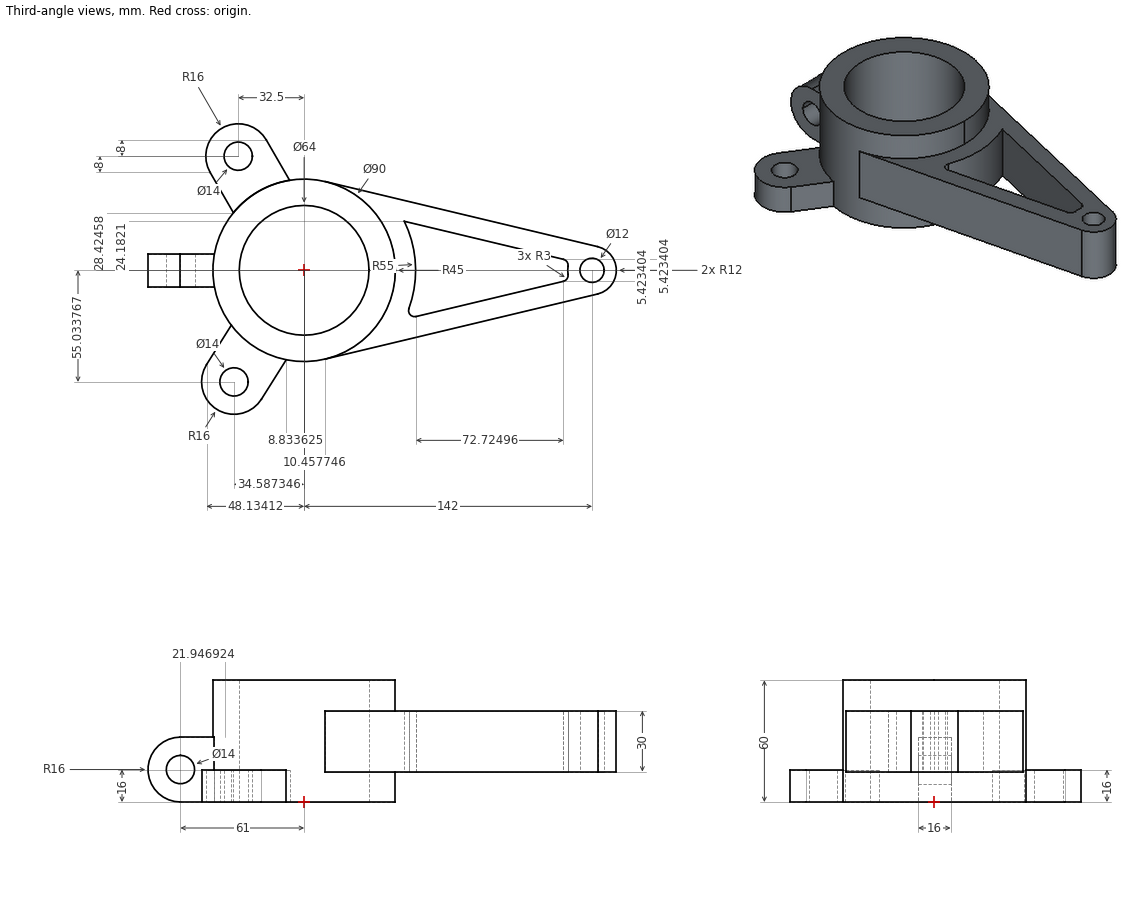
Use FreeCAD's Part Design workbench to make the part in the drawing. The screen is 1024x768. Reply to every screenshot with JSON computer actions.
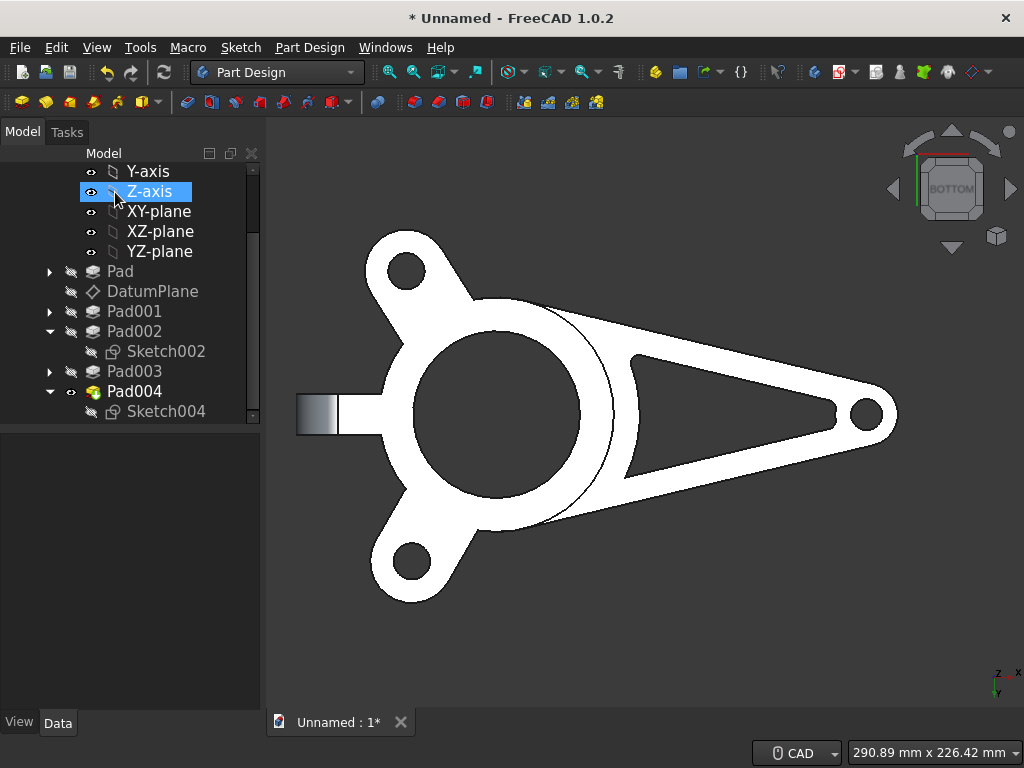
{"action": "key", "text": "4"}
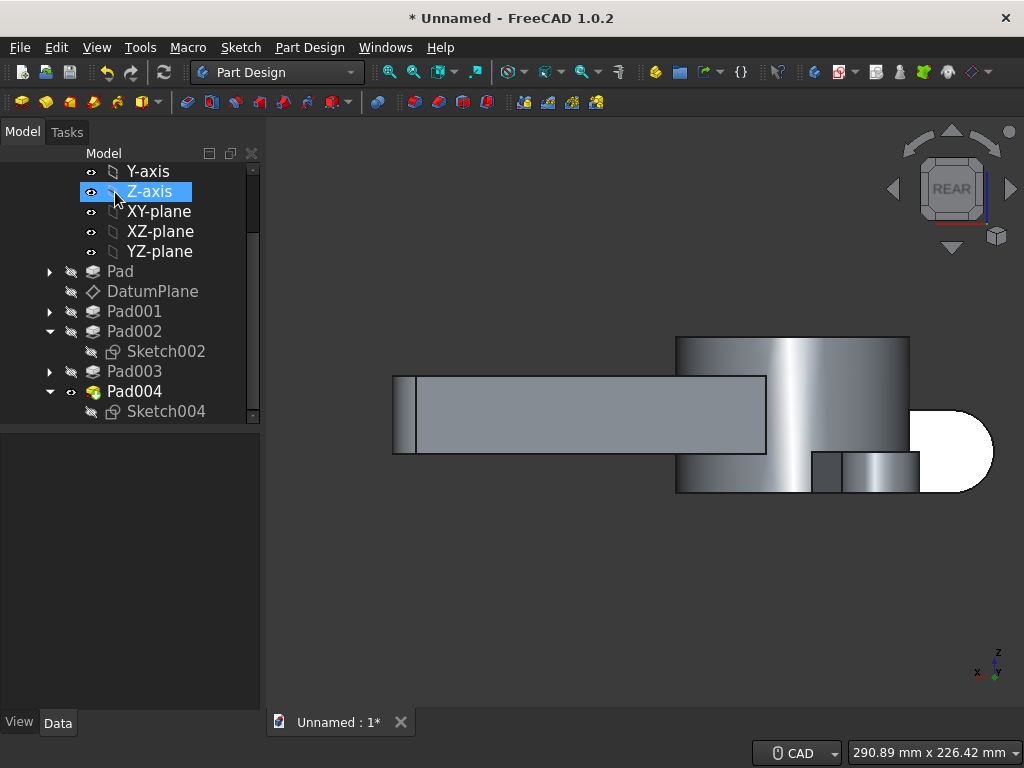
{"action": "left_click", "coordinate": [951, 451]}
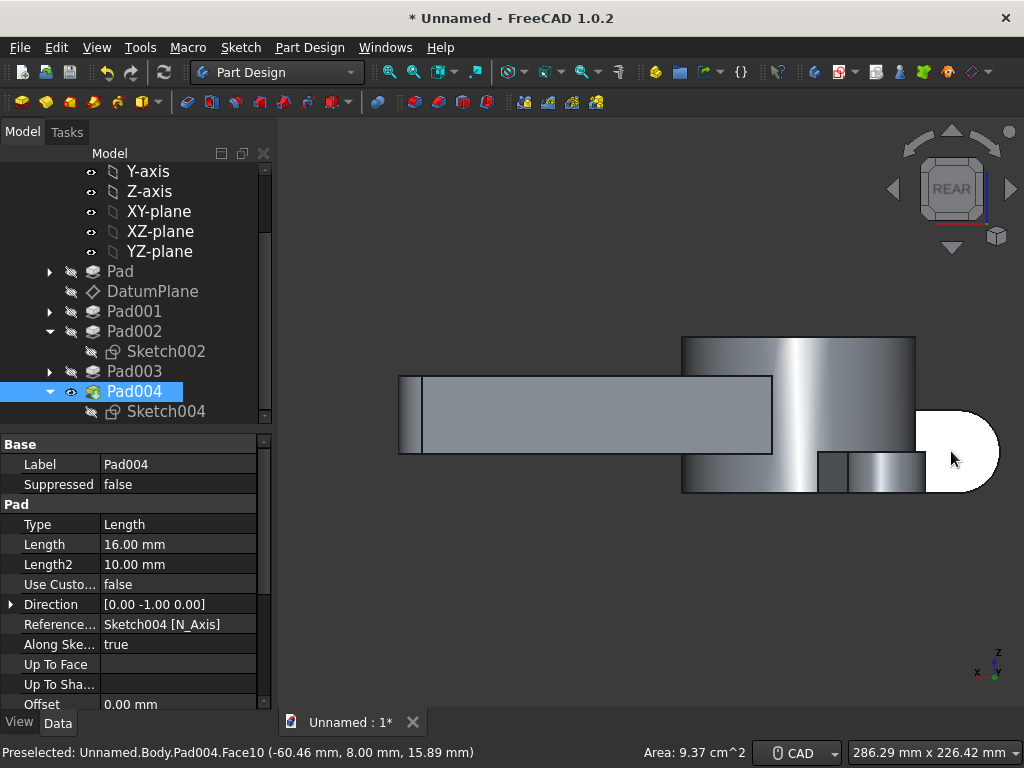
{"action": "left_click", "coordinate": [840, 72]}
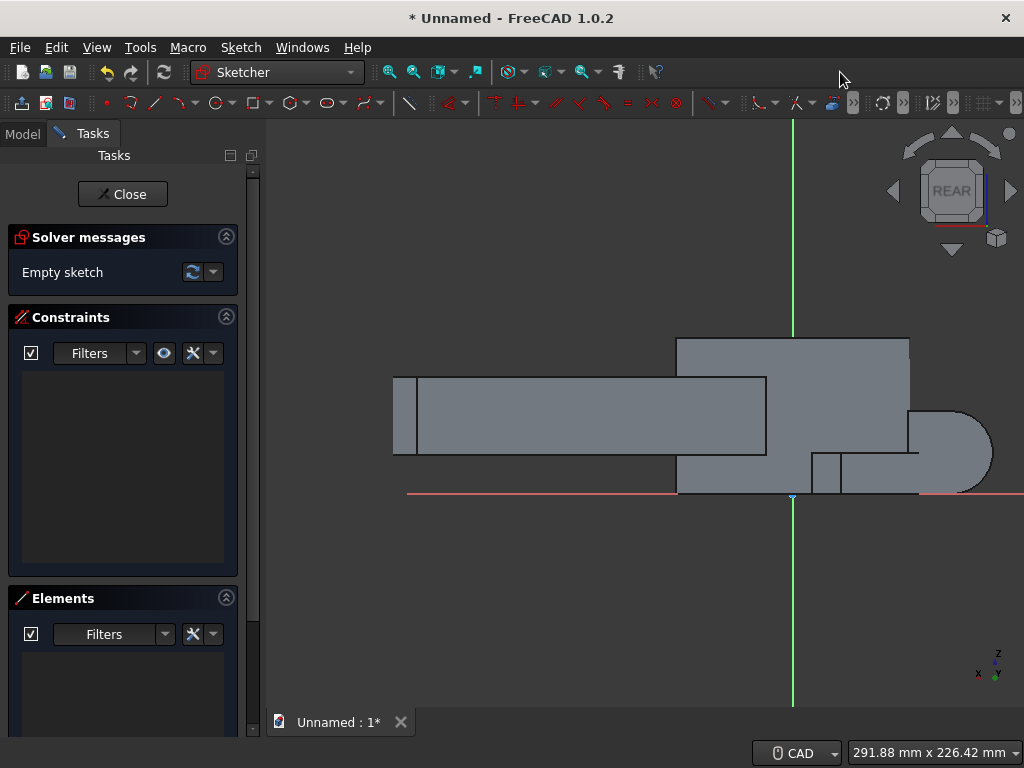
{"action": "scroll", "coordinate": [576, 413], "scroll_direction": "down", "scroll_amount": 5}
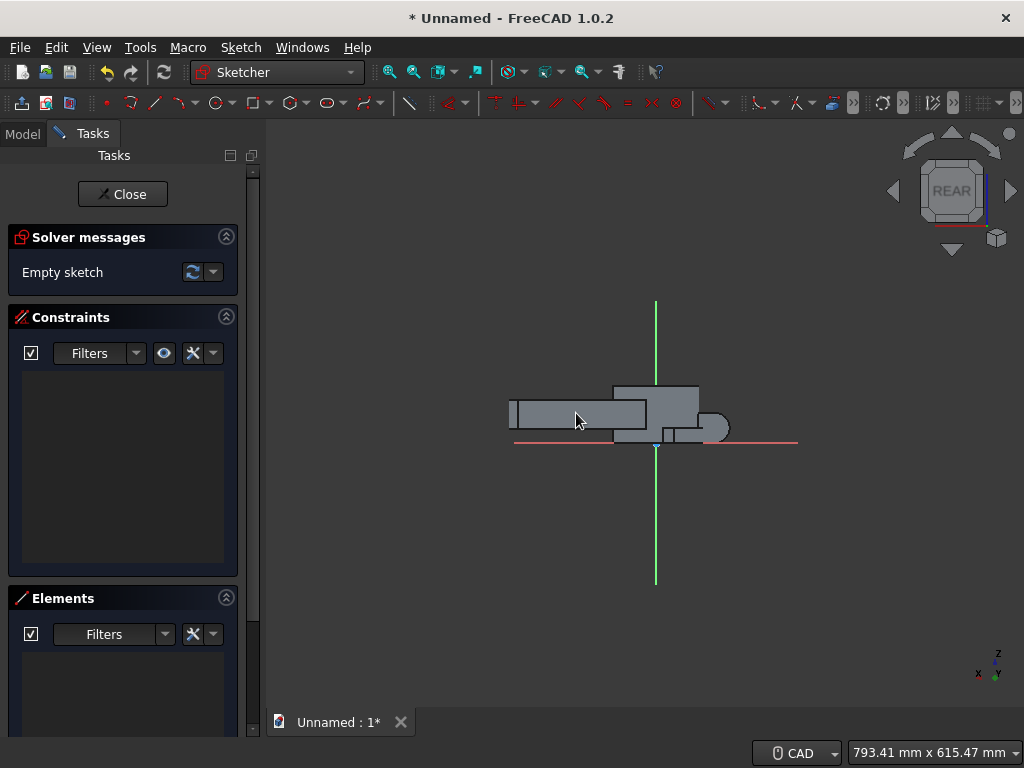
{"action": "scroll", "coordinate": [722, 429], "scroll_direction": "up", "scroll_amount": 15}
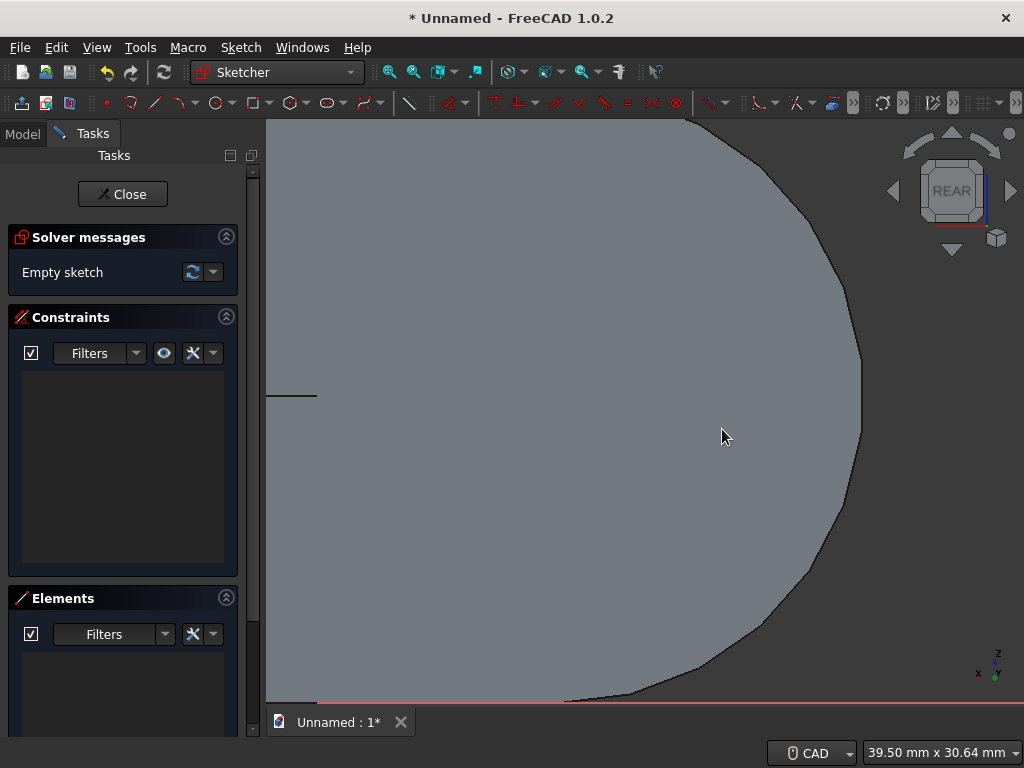
{"action": "scroll", "coordinate": [517, 362], "scroll_direction": "up", "scroll_amount": 2}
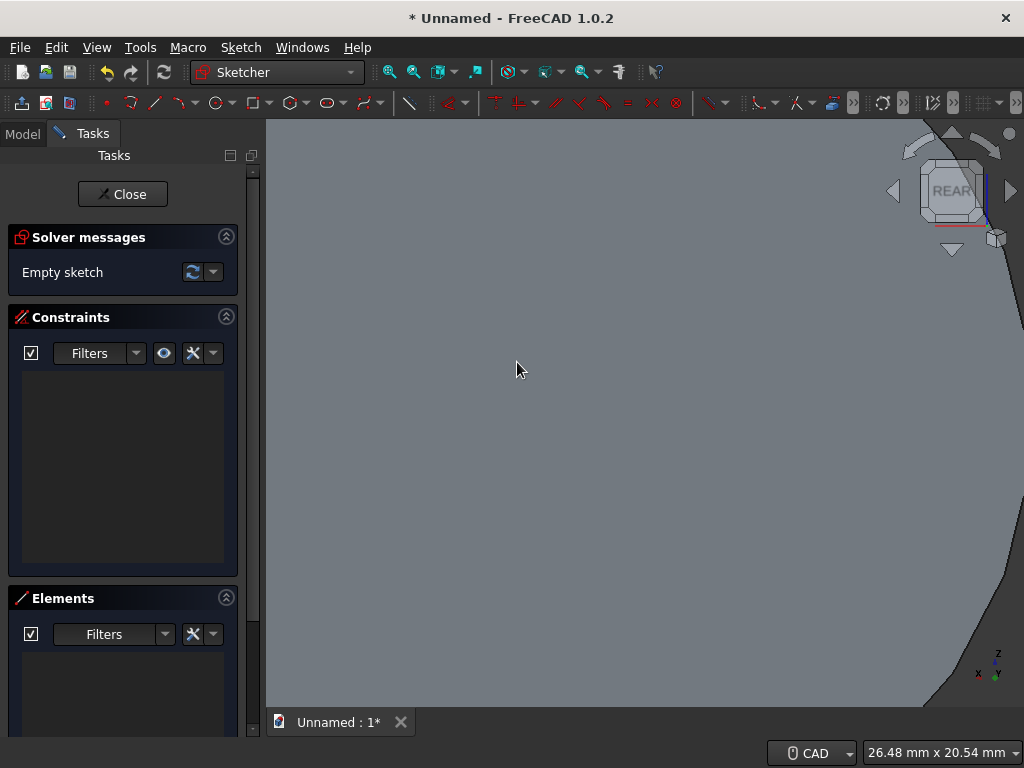
{"action": "key", "text": "g c"}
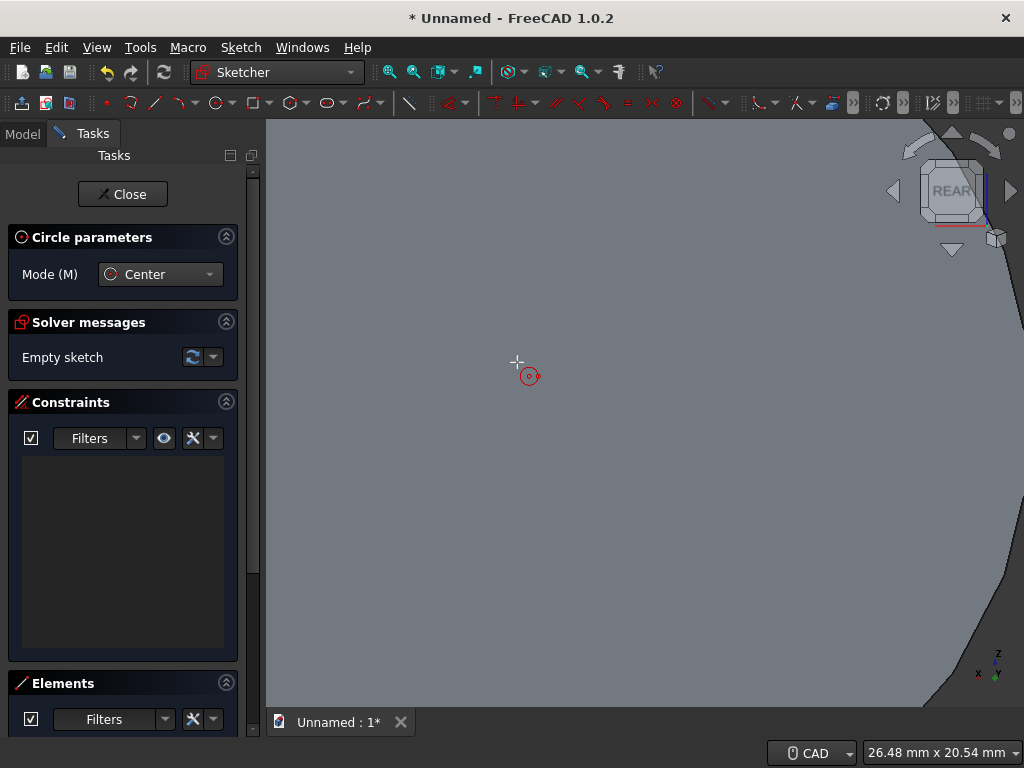
{"action": "left_click", "coordinate": [576, 413]}
{"action": "left_click", "coordinate": [718, 271]}
{"action": "key", "text": "Escape"}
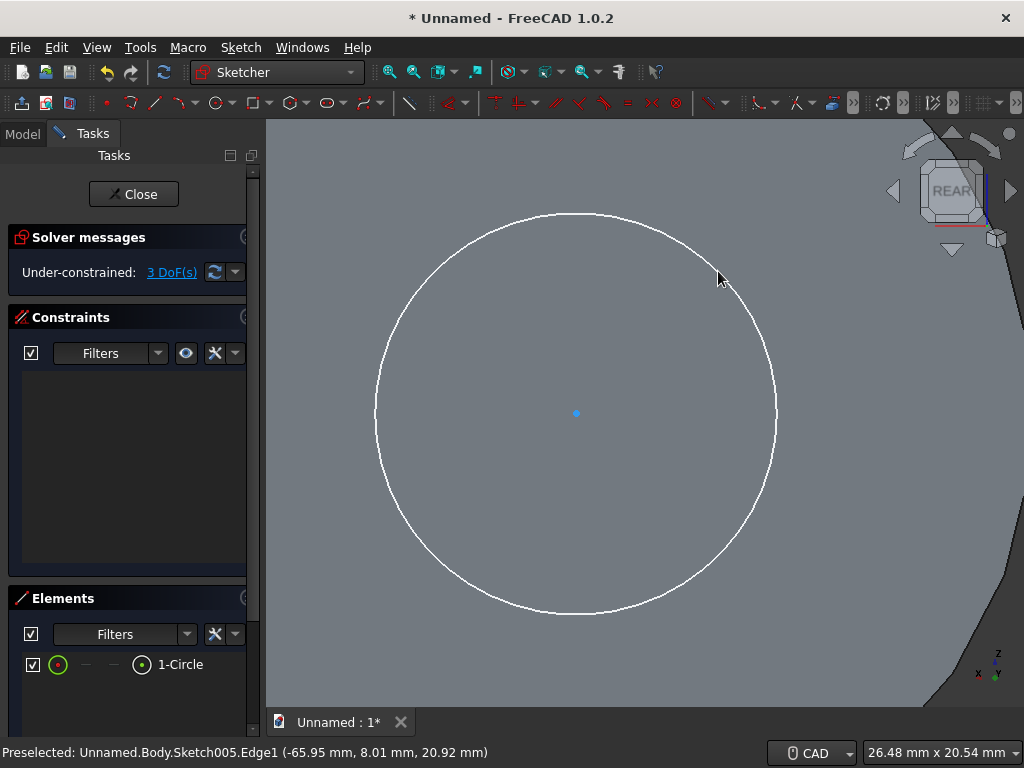
{"action": "left_click", "coordinate": [448, 104]}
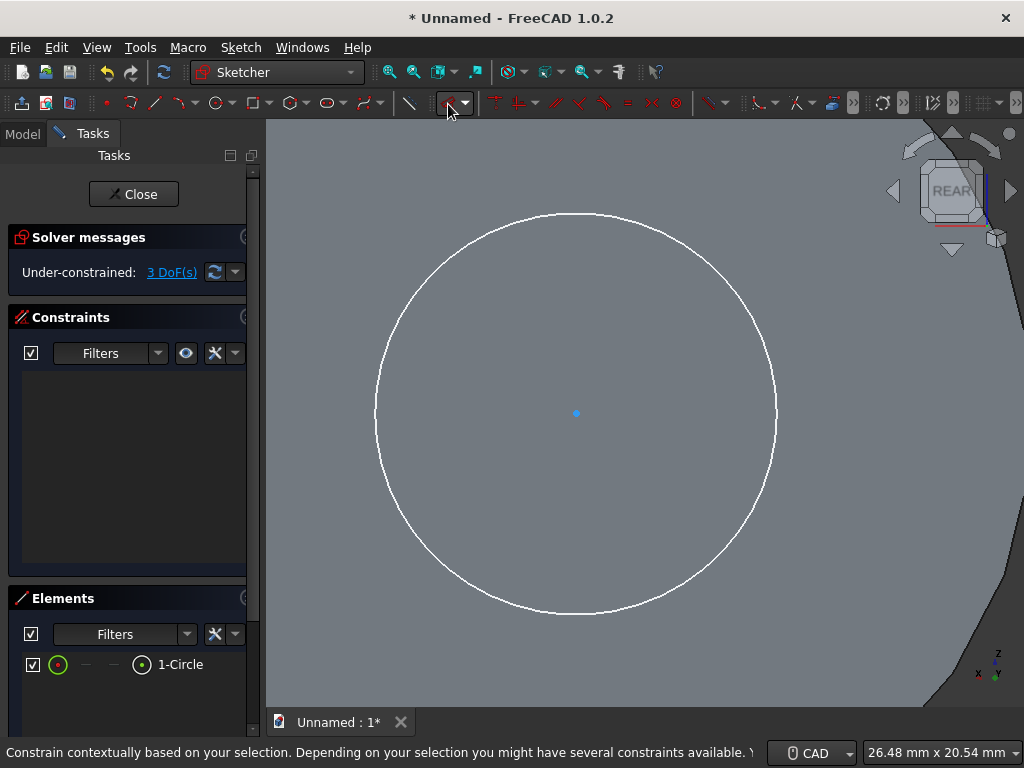
{"action": "left_click", "coordinate": [718, 272]}
{"action": "left_click", "coordinate": [741, 249]}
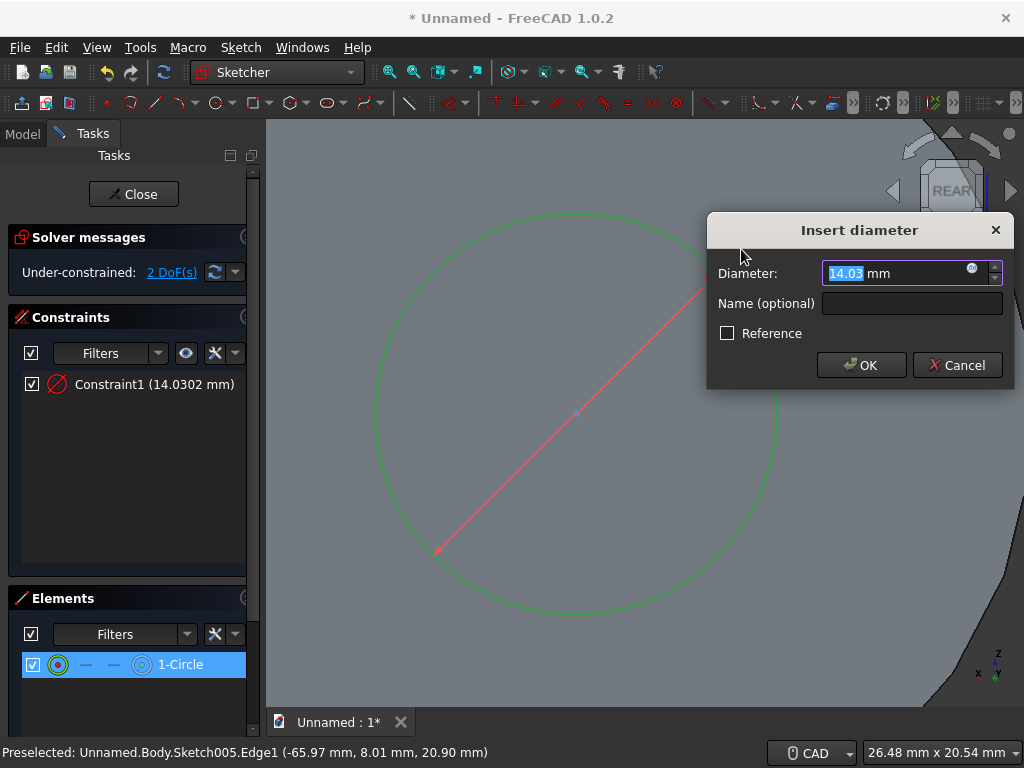
{"action": "type", "text": "14"}
{"action": "key", "text": "Return"}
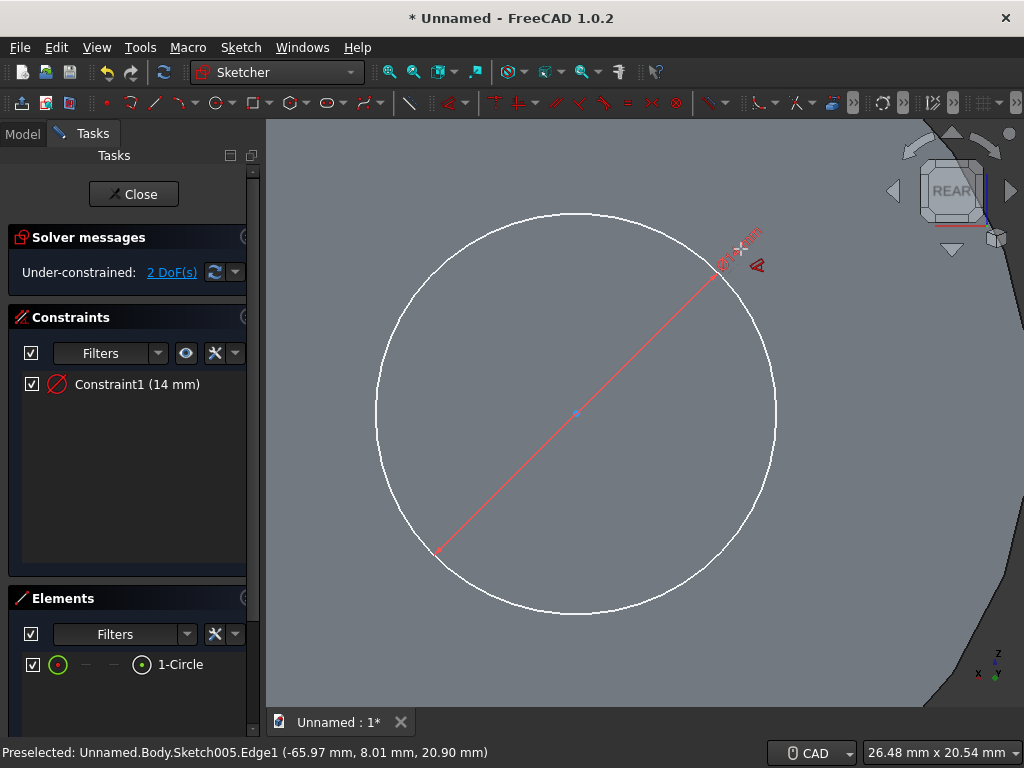
{"action": "left_click", "coordinate": [576, 414]}
{"action": "left_click", "coordinate": [435, 380]}